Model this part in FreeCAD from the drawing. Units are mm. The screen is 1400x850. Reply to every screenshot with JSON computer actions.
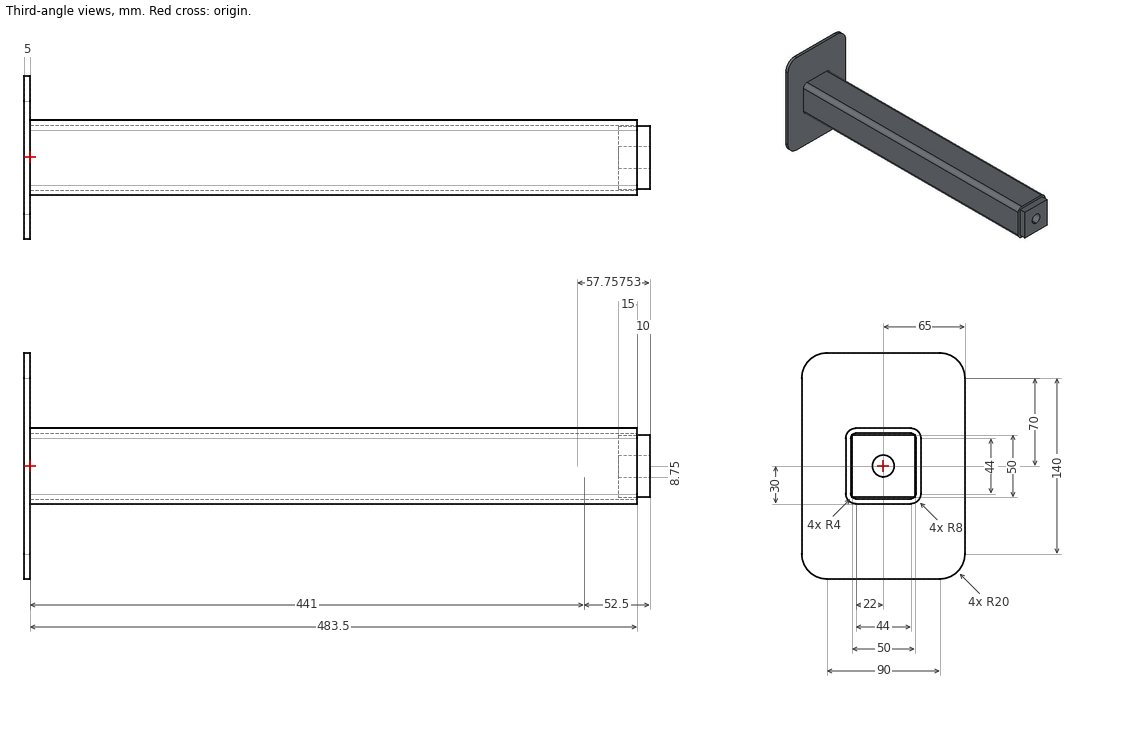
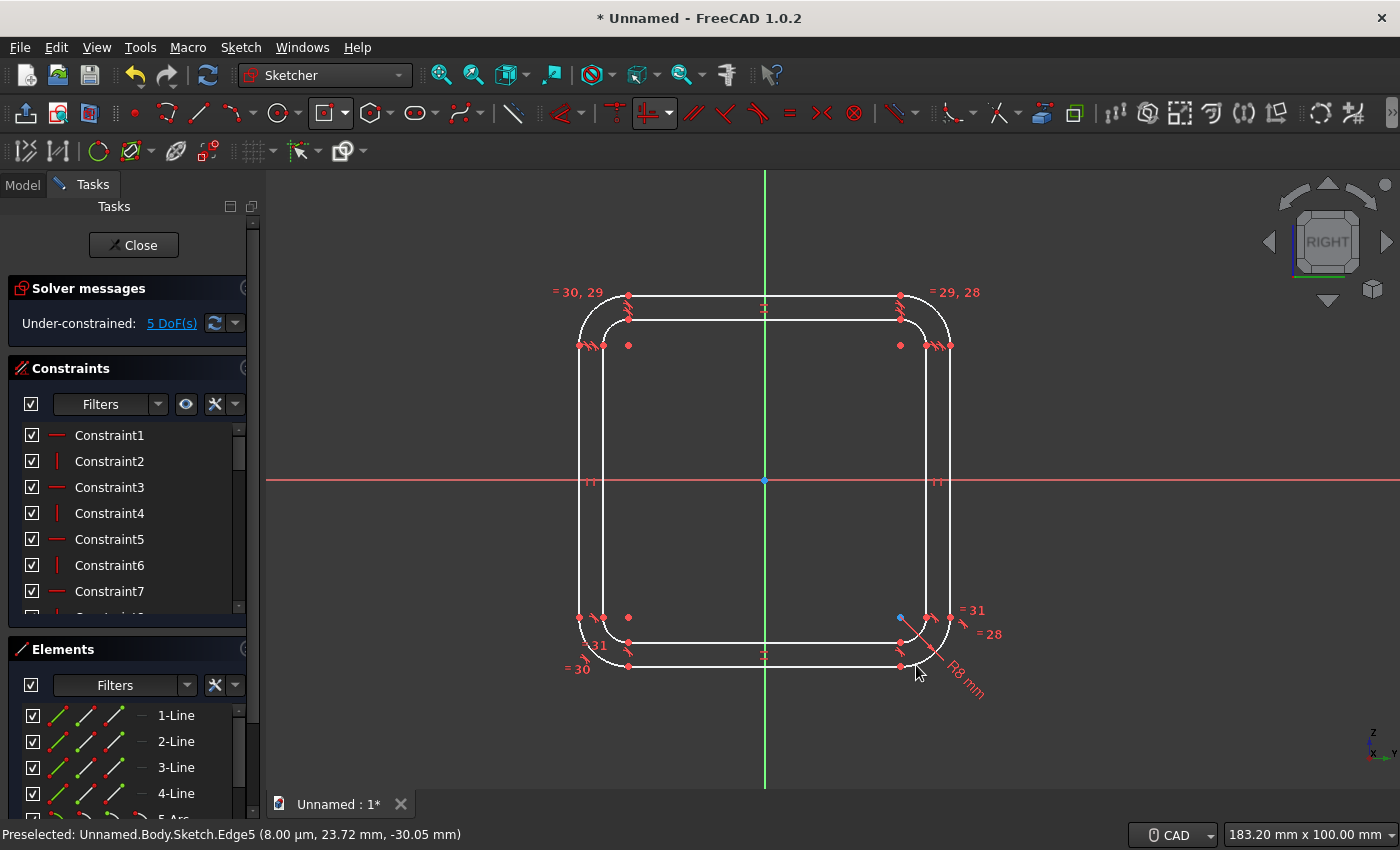
{"action": "scroll", "coordinate": [606, 629], "scroll_direction": "up", "scroll_amount": 3}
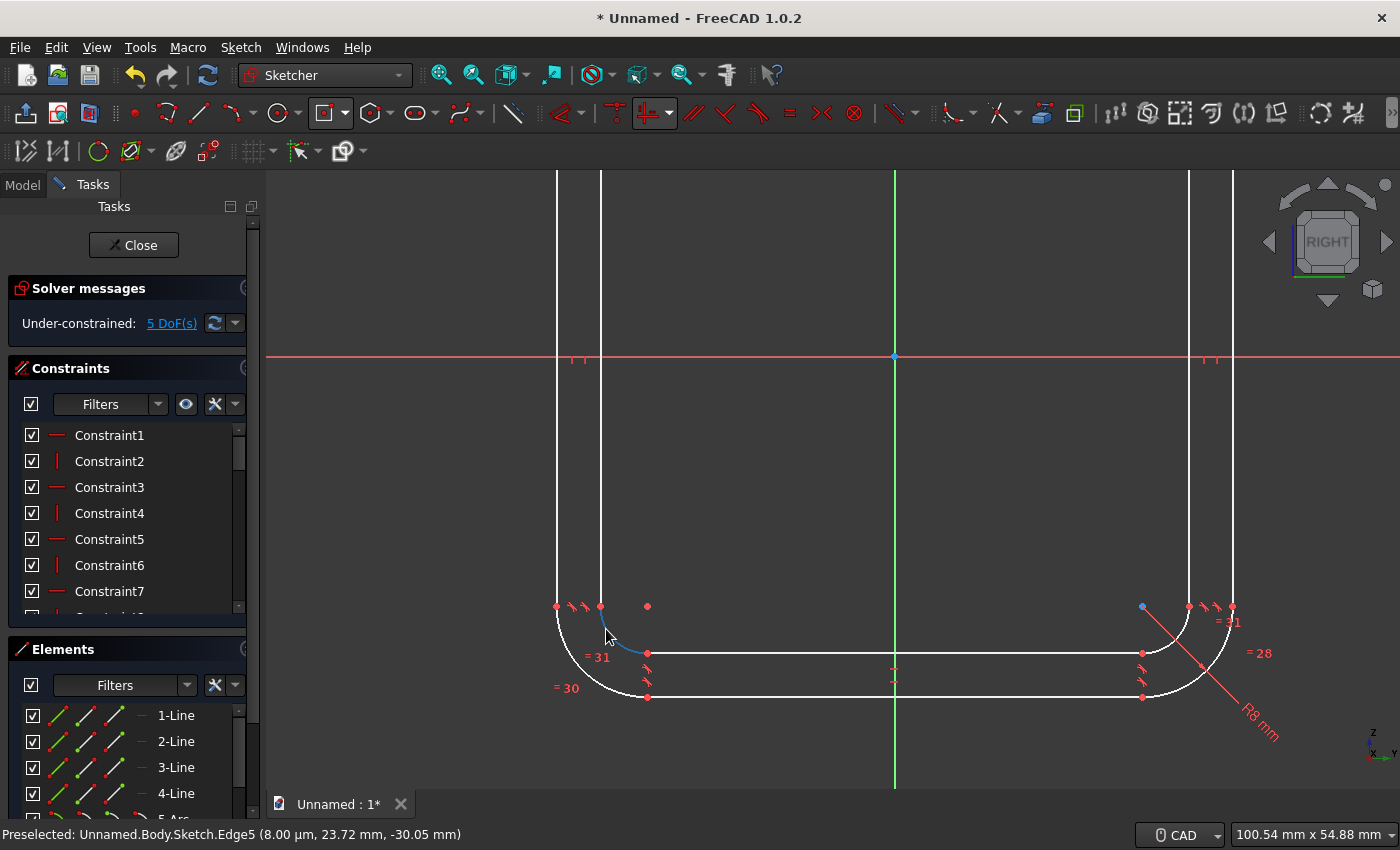
{"action": "left_click", "coordinate": [606, 628]}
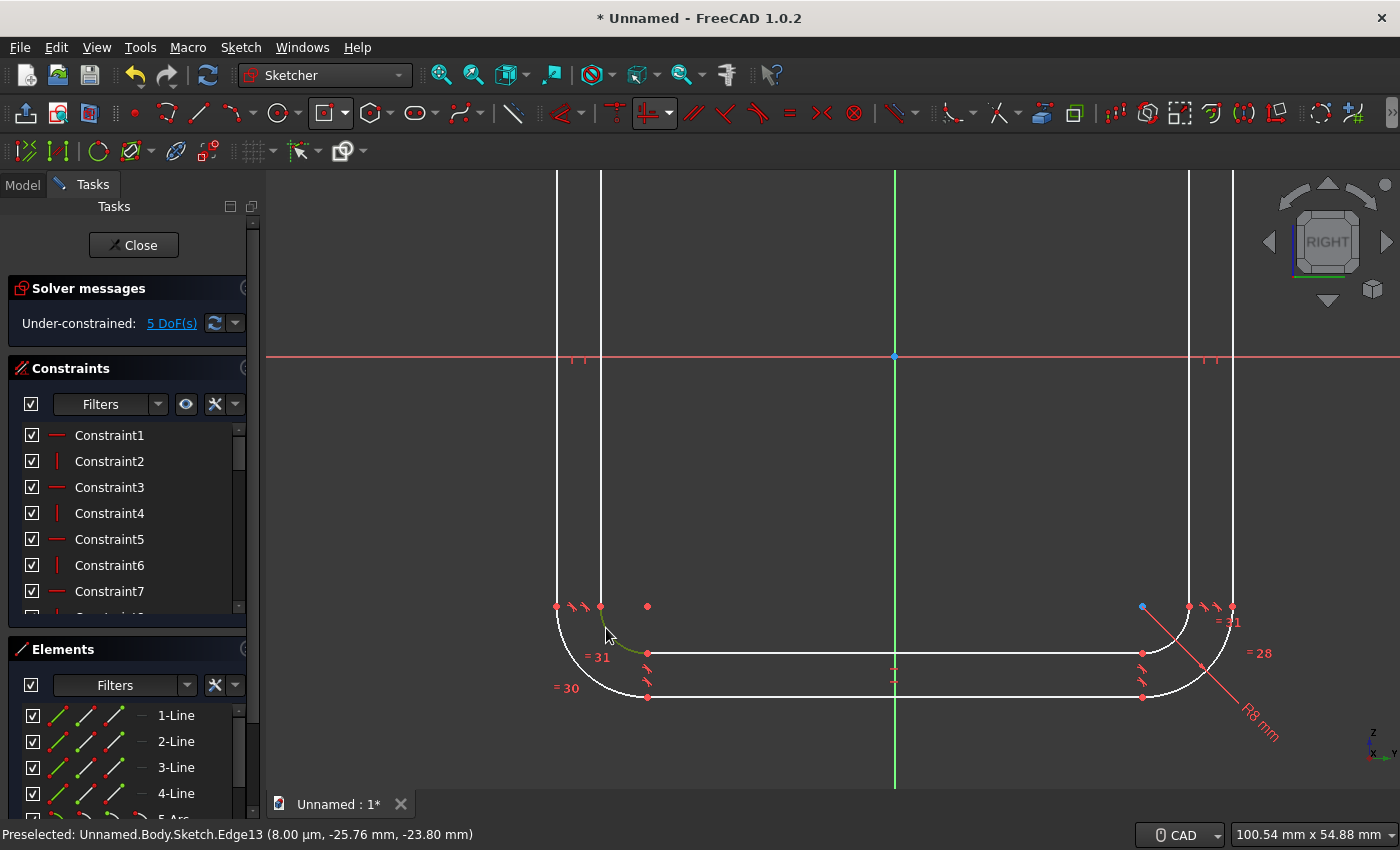
{"action": "key", "text": "k r"}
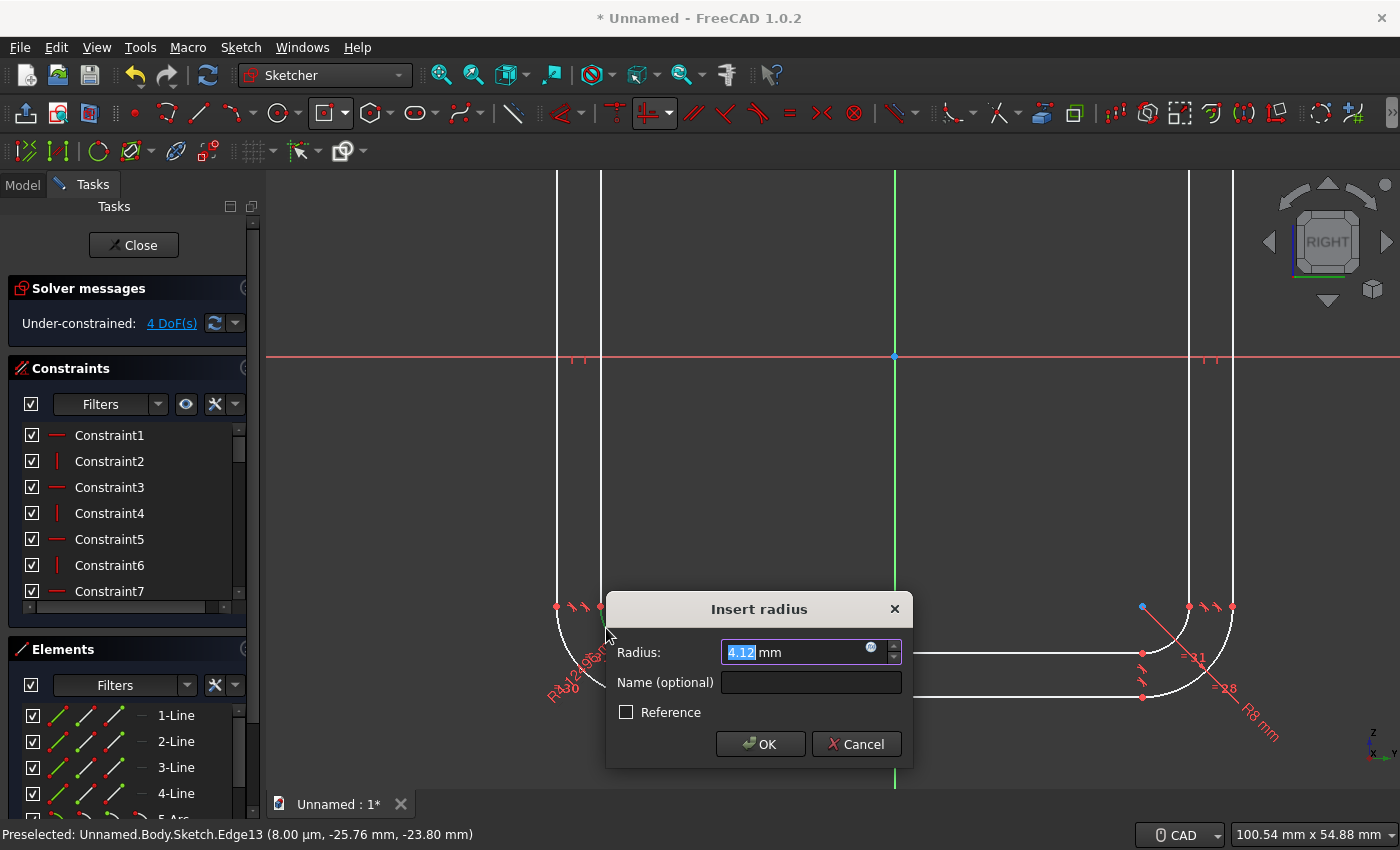
{"action": "type", "text": "4"}
{"action": "key", "text": "Return"}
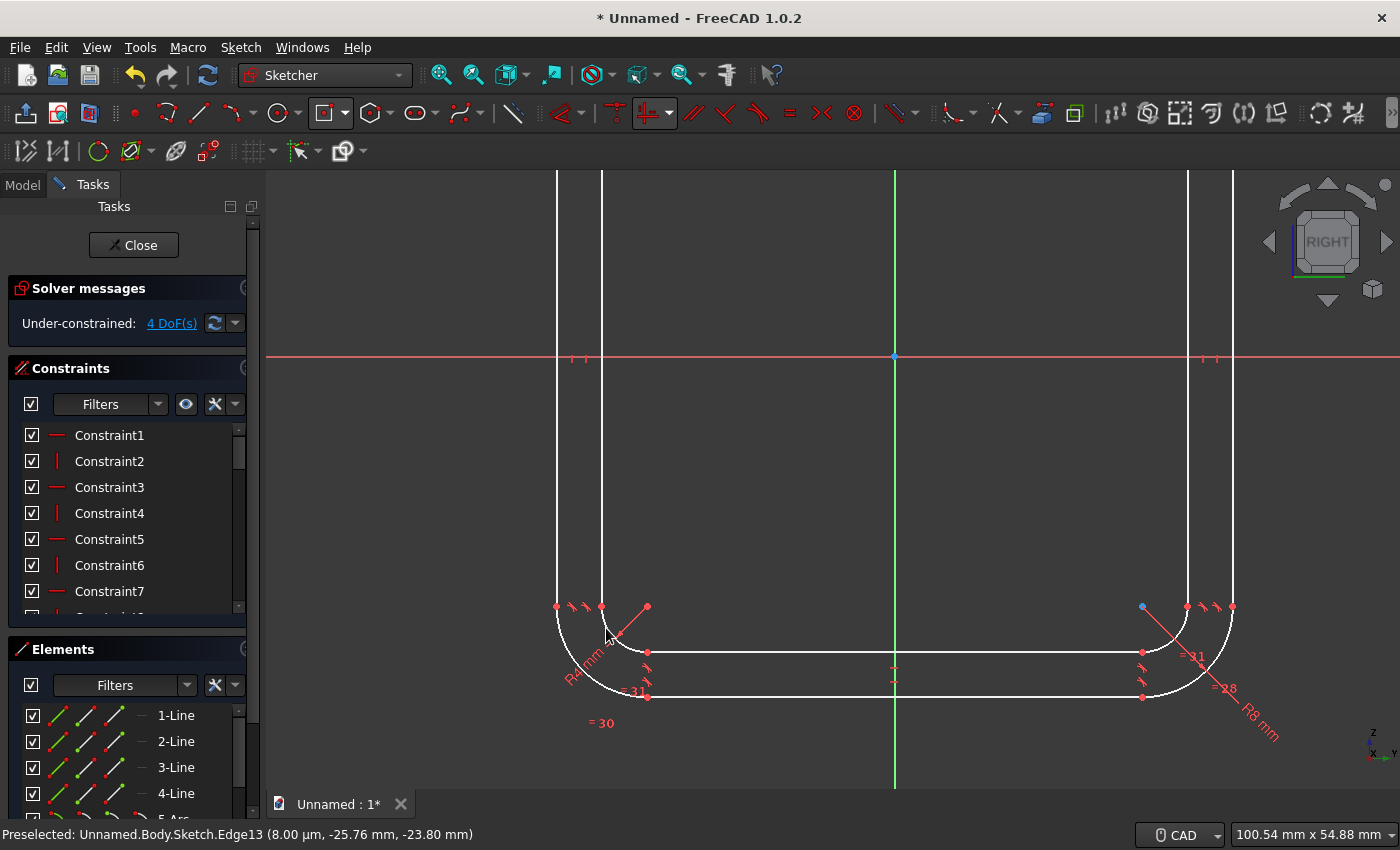
{"action": "left_click", "coordinate": [796, 697]}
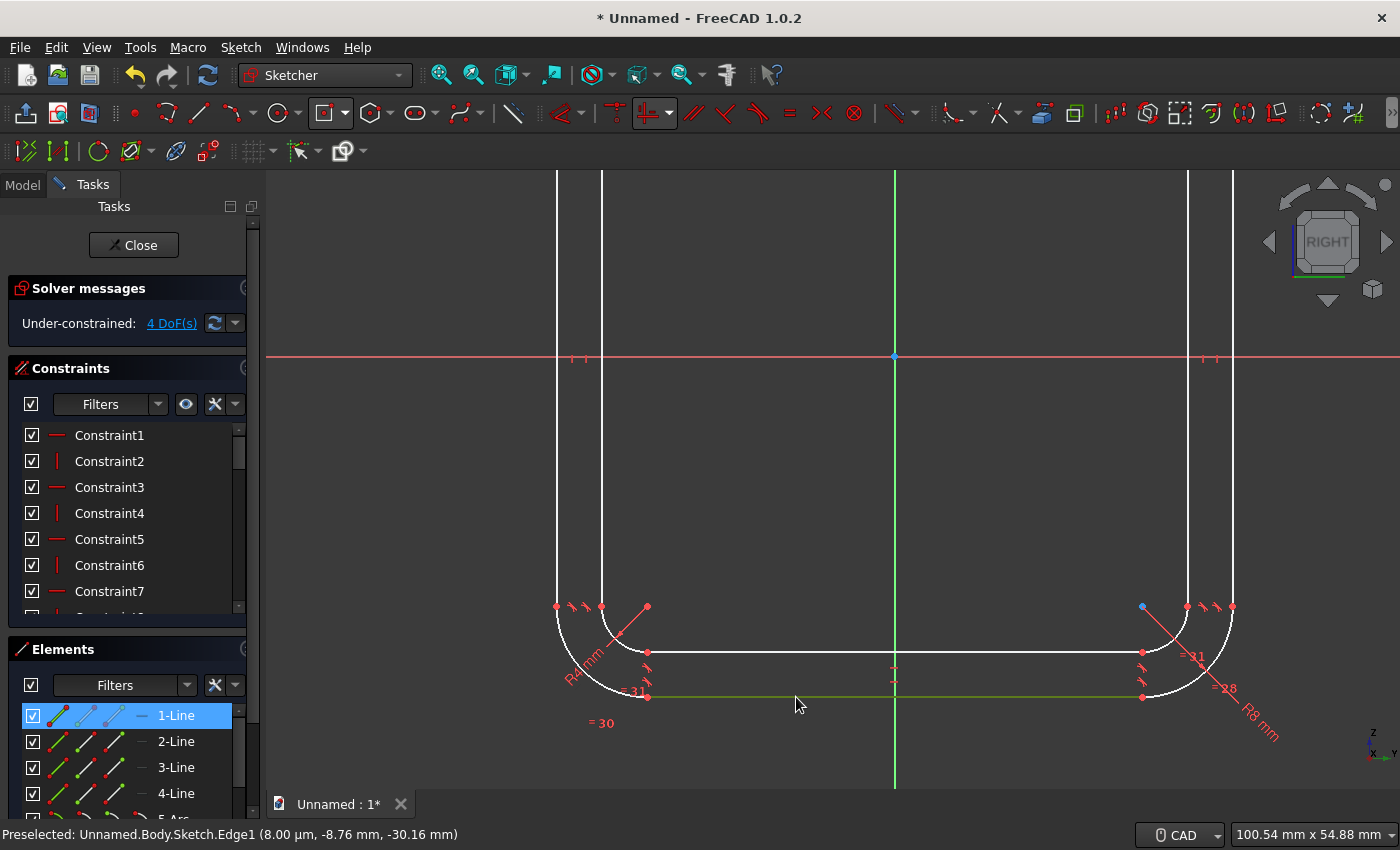
{"action": "key", "text": "l"}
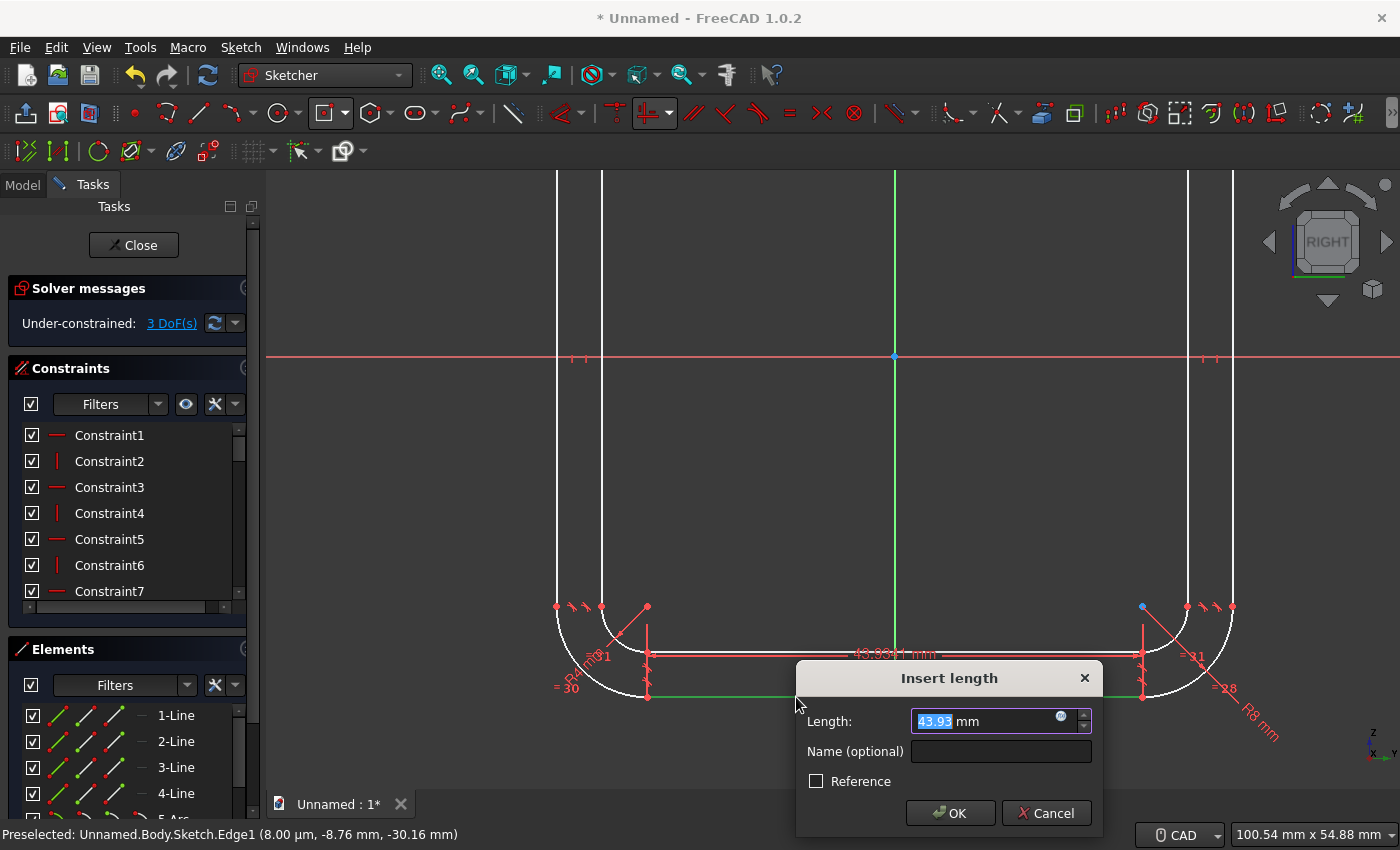
{"action": "type", "text": "44"}
{"action": "key", "text": "Return"}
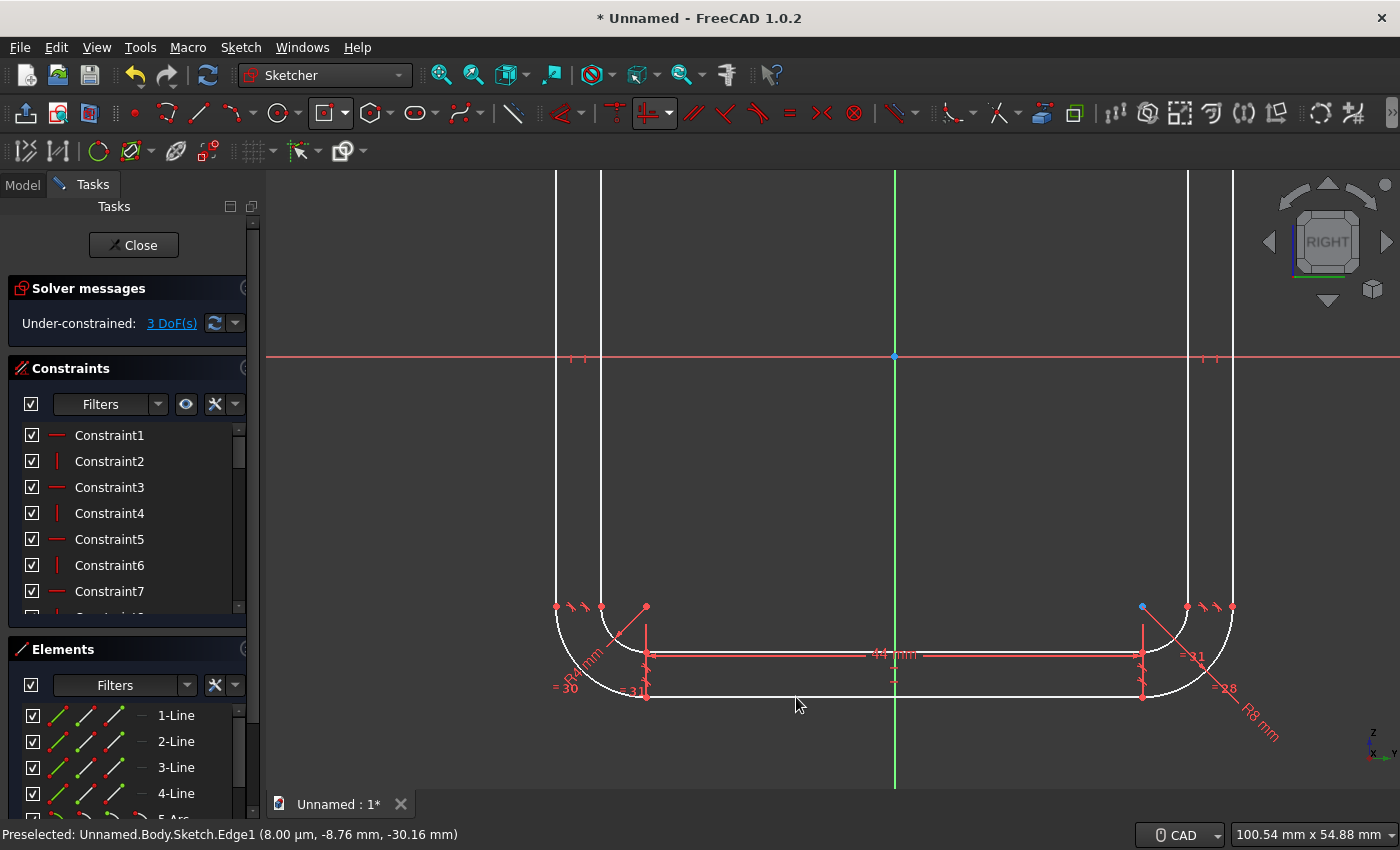
{"action": "left_click", "coordinate": [1233, 458]}